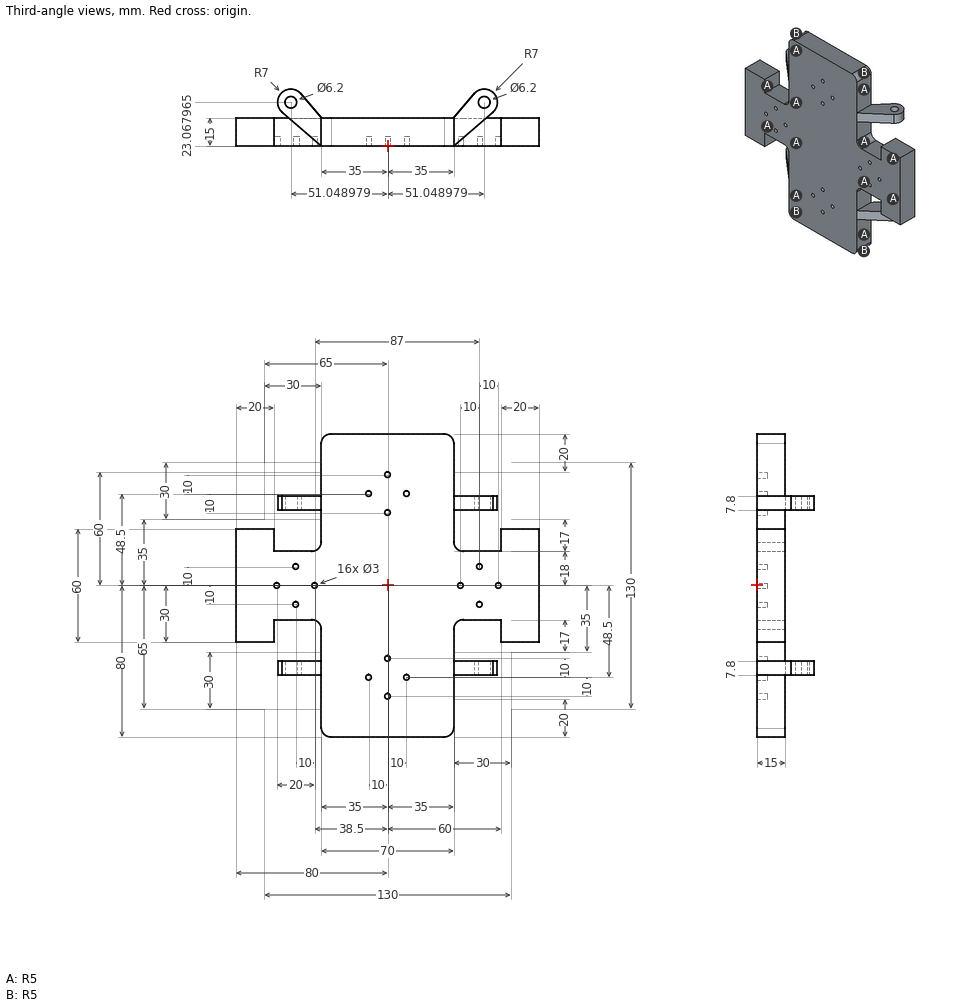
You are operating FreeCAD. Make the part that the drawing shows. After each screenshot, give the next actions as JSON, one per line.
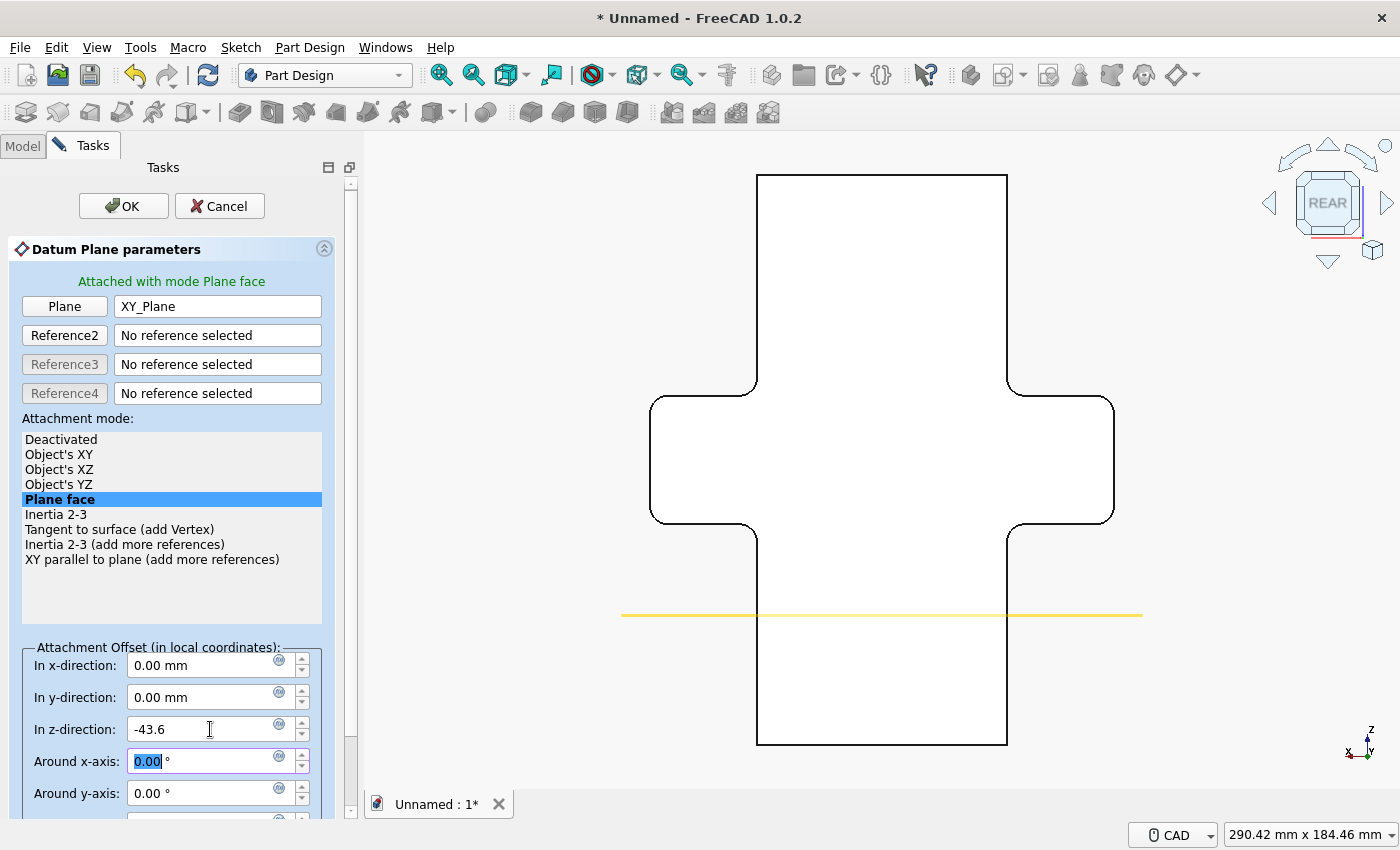
{"action": "left_click", "coordinate": [124, 206]}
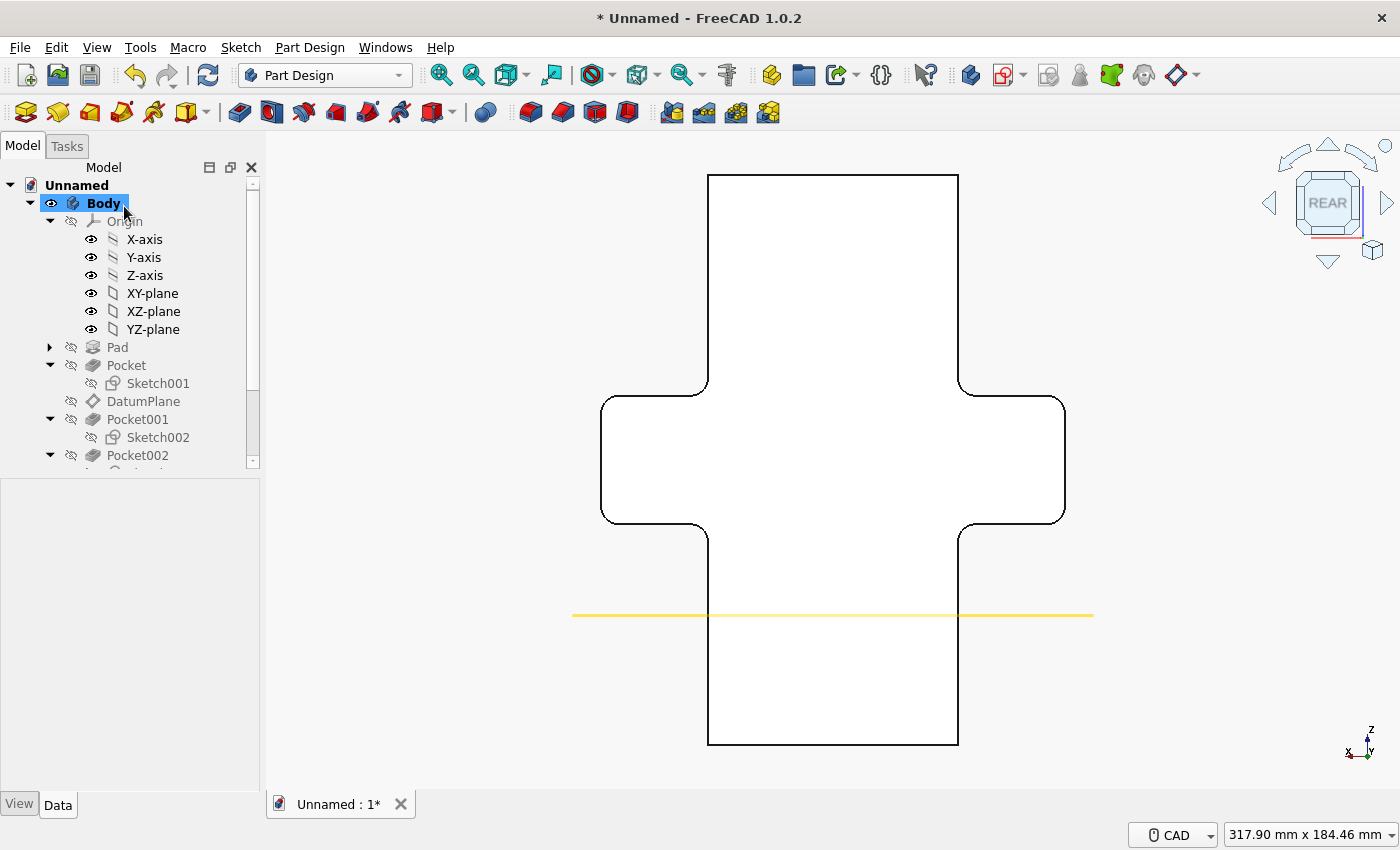
{"action": "scroll", "coordinate": [100, 325], "scroll_direction": "down", "scroll_amount": 3}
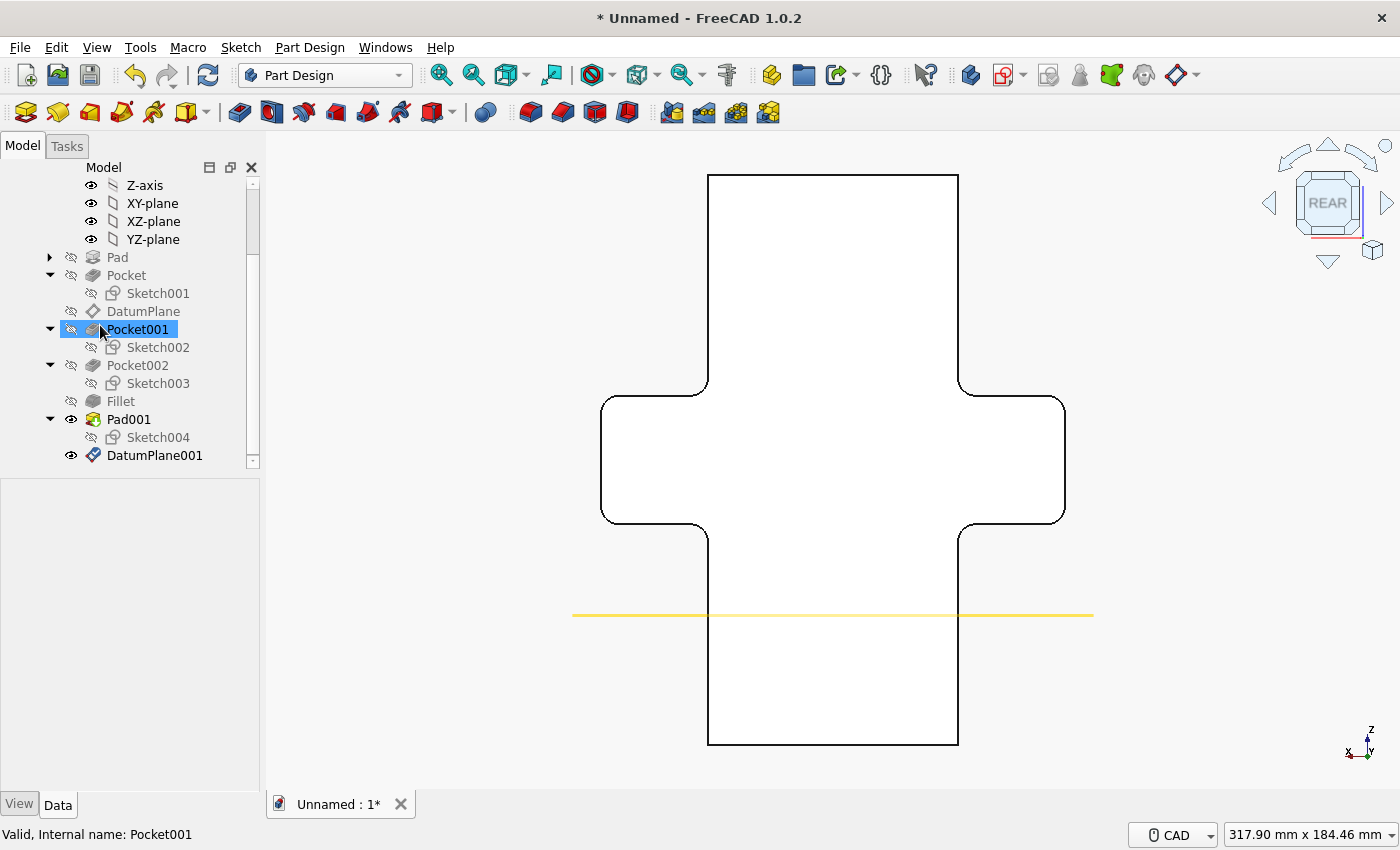
{"action": "left_click", "coordinate": [116, 455]}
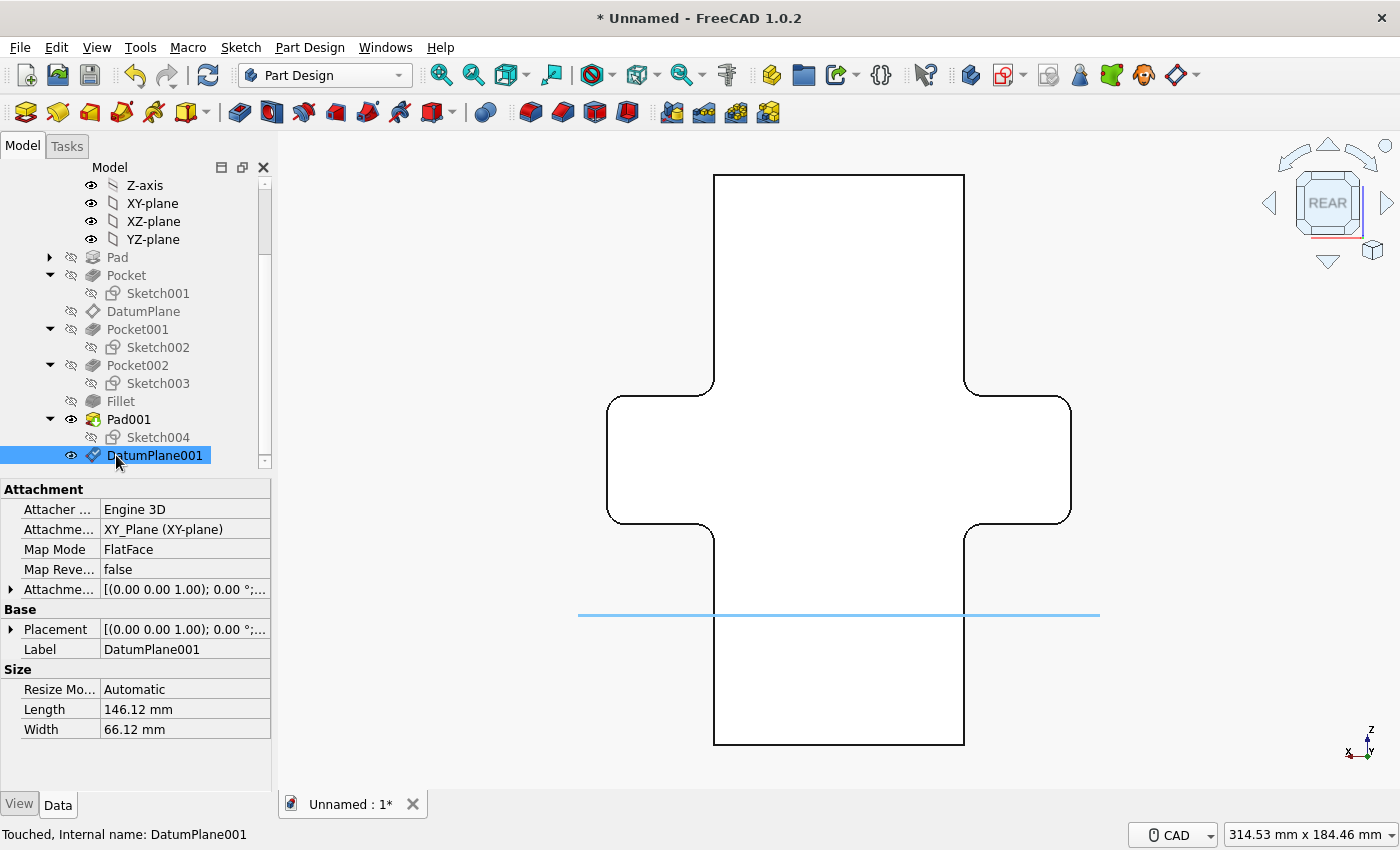
{"action": "left_click", "coordinate": [1004, 76]}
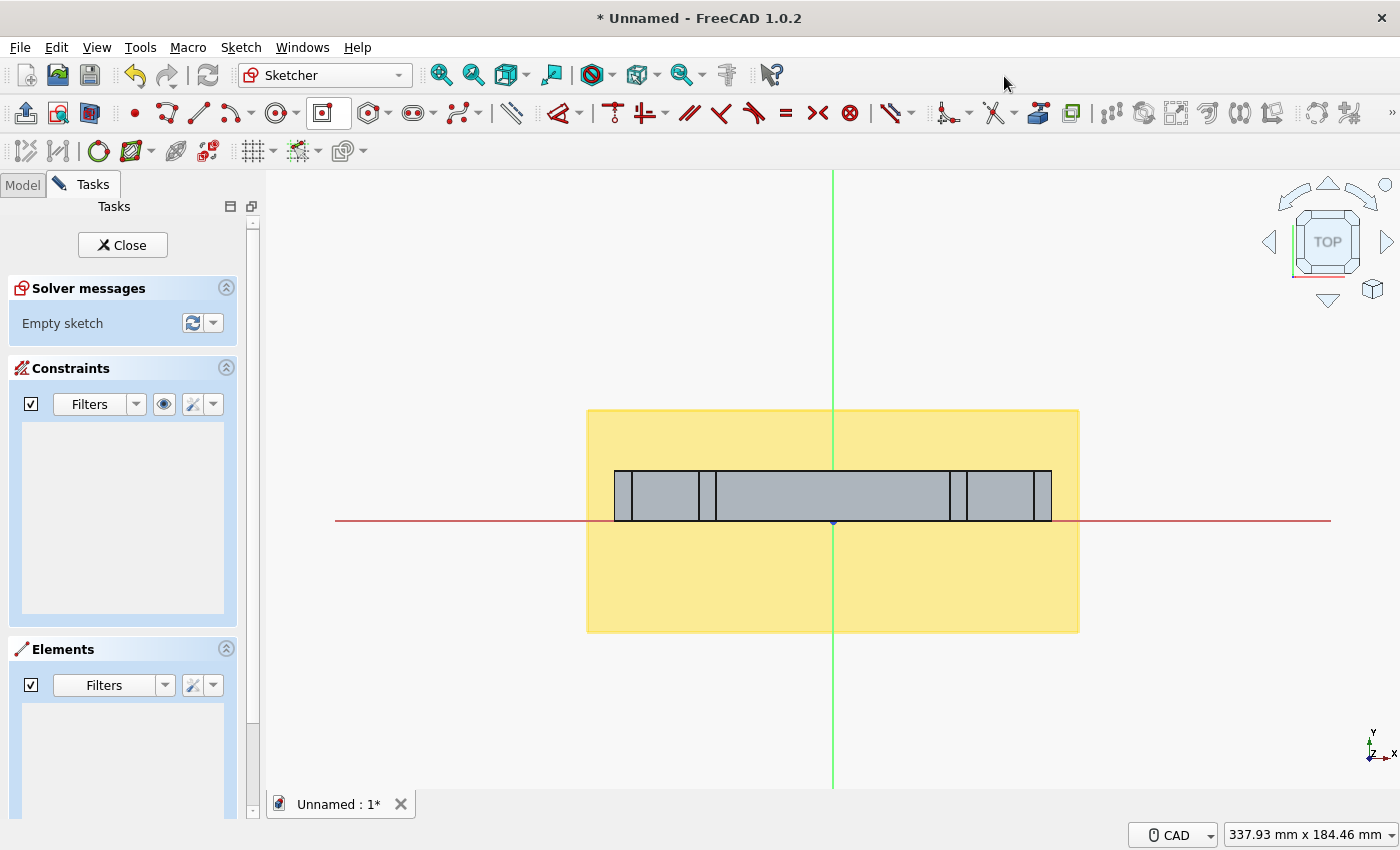
{"action": "left_click", "coordinate": [90, 114]}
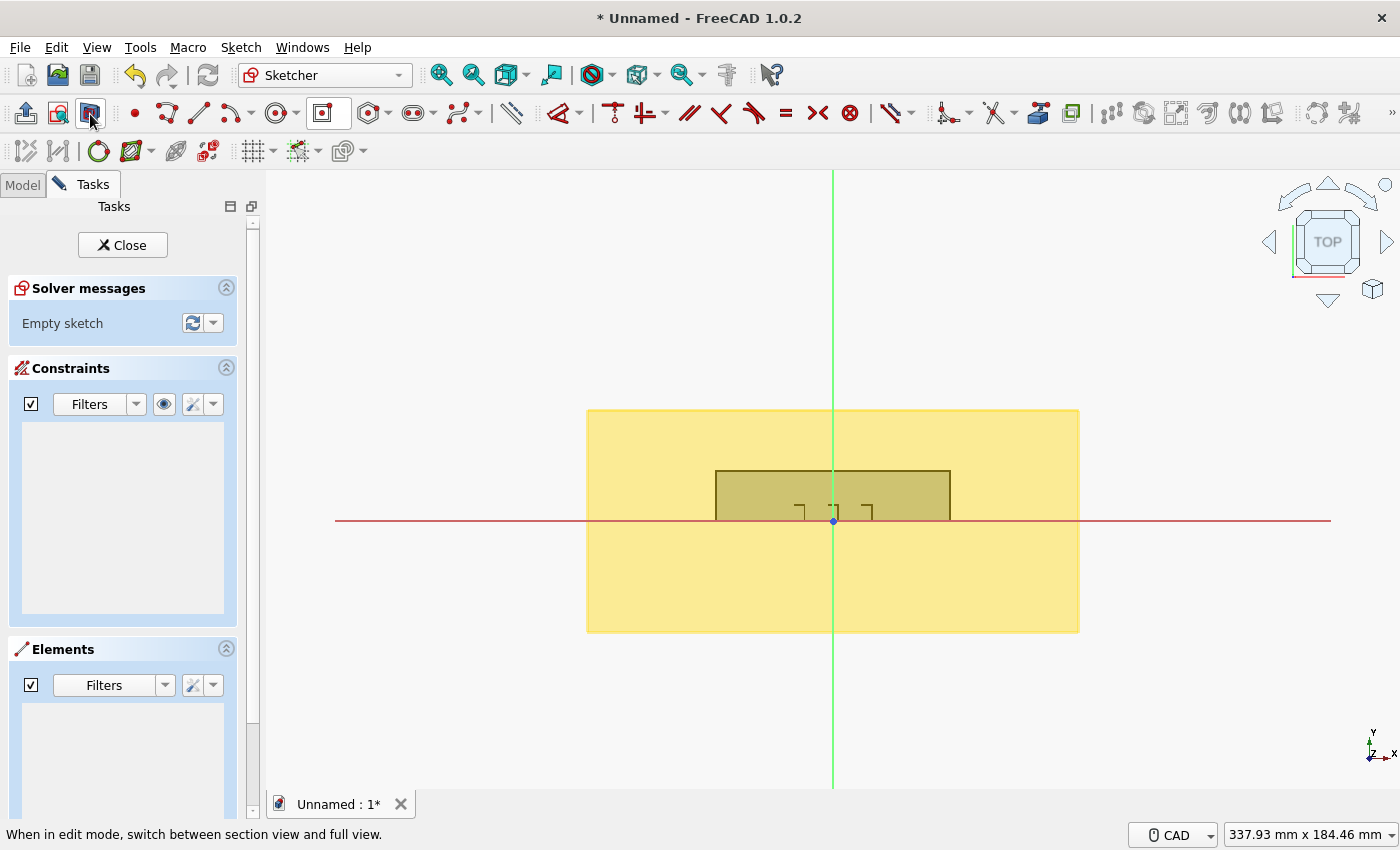
{"action": "scroll", "coordinate": [728, 472], "scroll_direction": "up", "scroll_amount": 6}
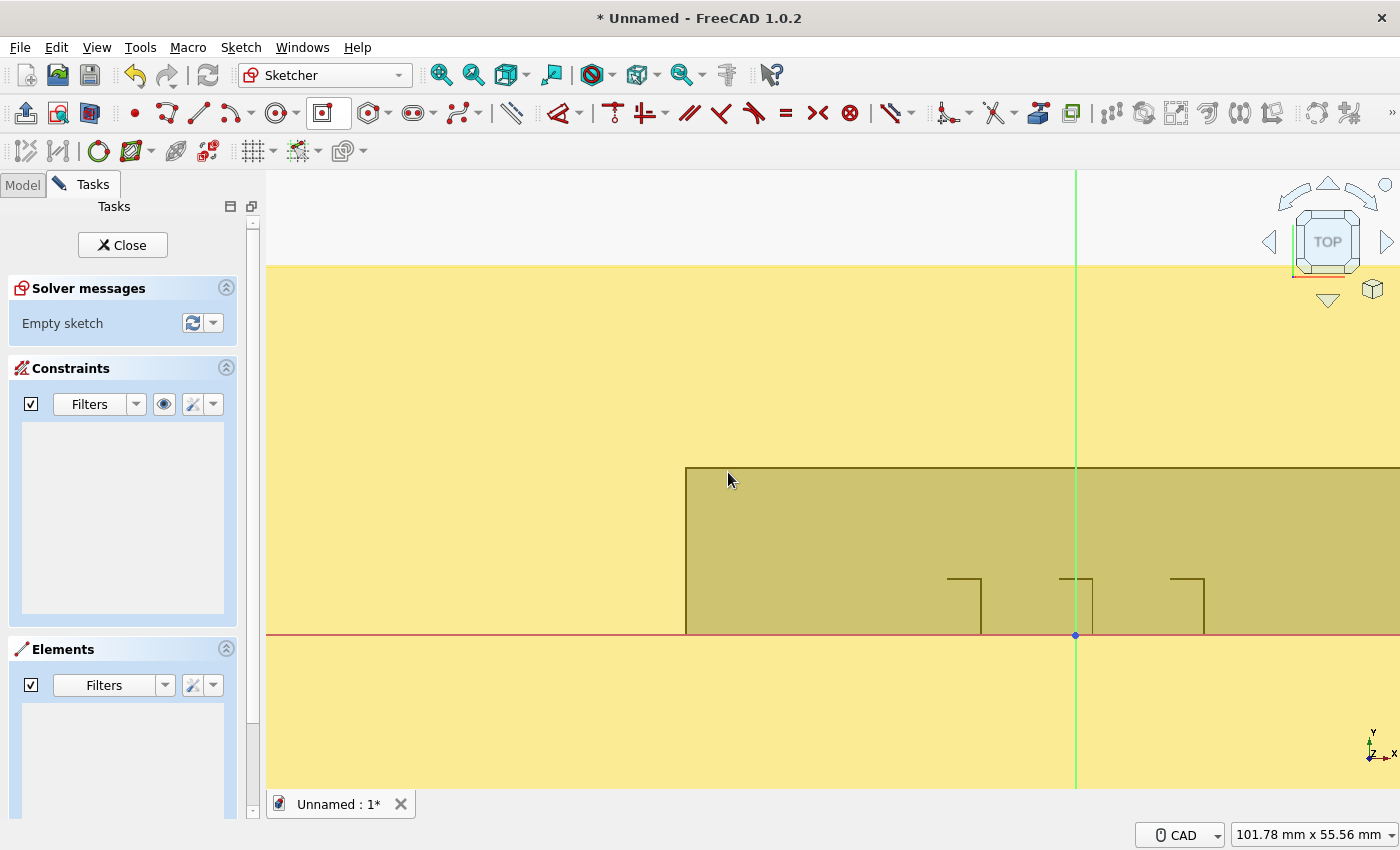
{"action": "key", "text": "g m"}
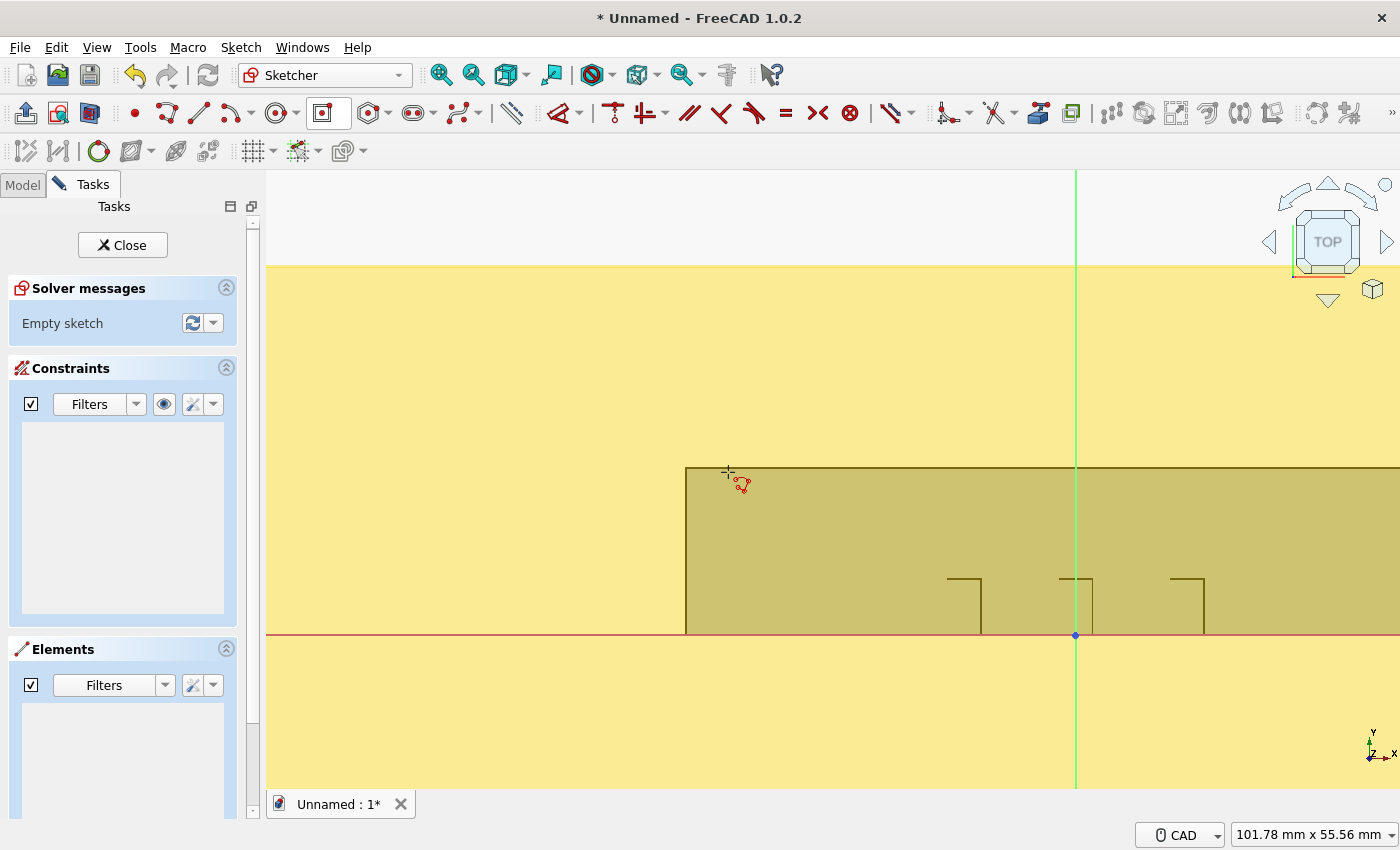
{"action": "left_click", "coordinate": [566, 328]}
{"action": "left_click", "coordinate": [686, 468]}
{"action": "left_click", "coordinate": [686, 635]}
{"action": "left_click", "coordinate": [456, 437]}
{"action": "right_click", "coordinate": [456, 437]}